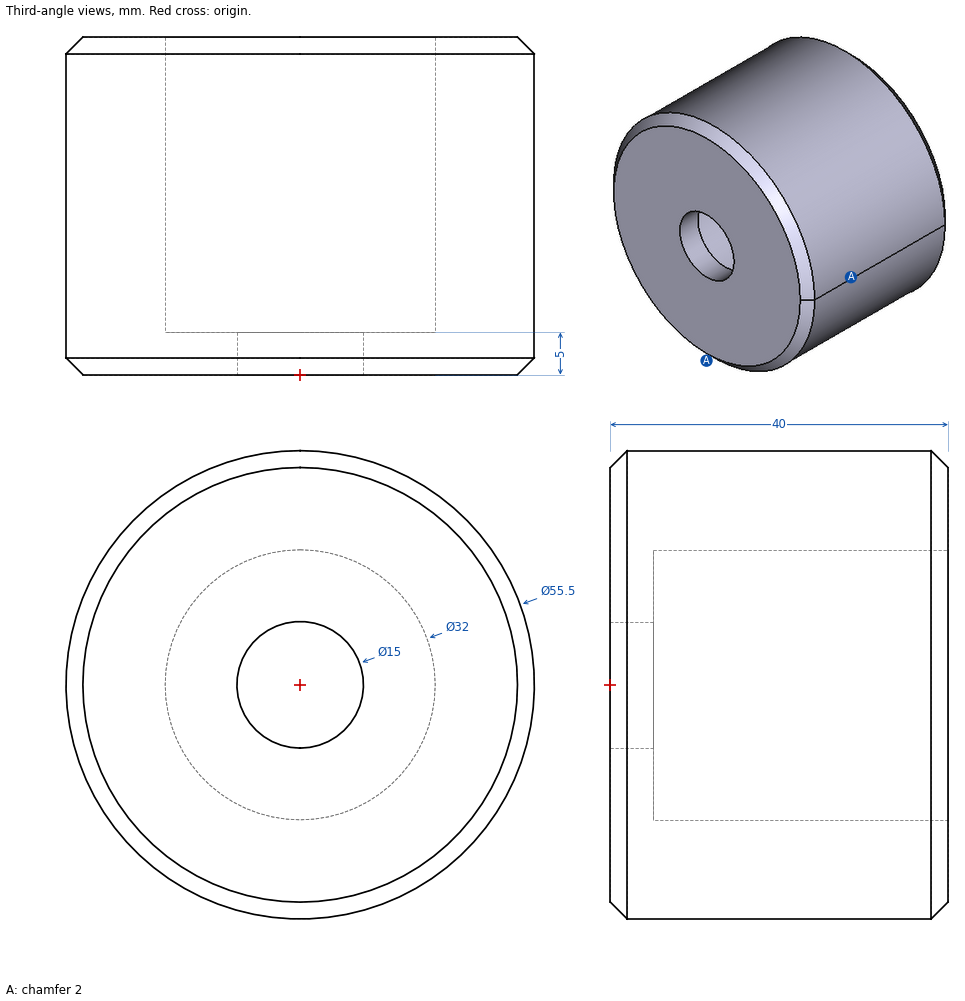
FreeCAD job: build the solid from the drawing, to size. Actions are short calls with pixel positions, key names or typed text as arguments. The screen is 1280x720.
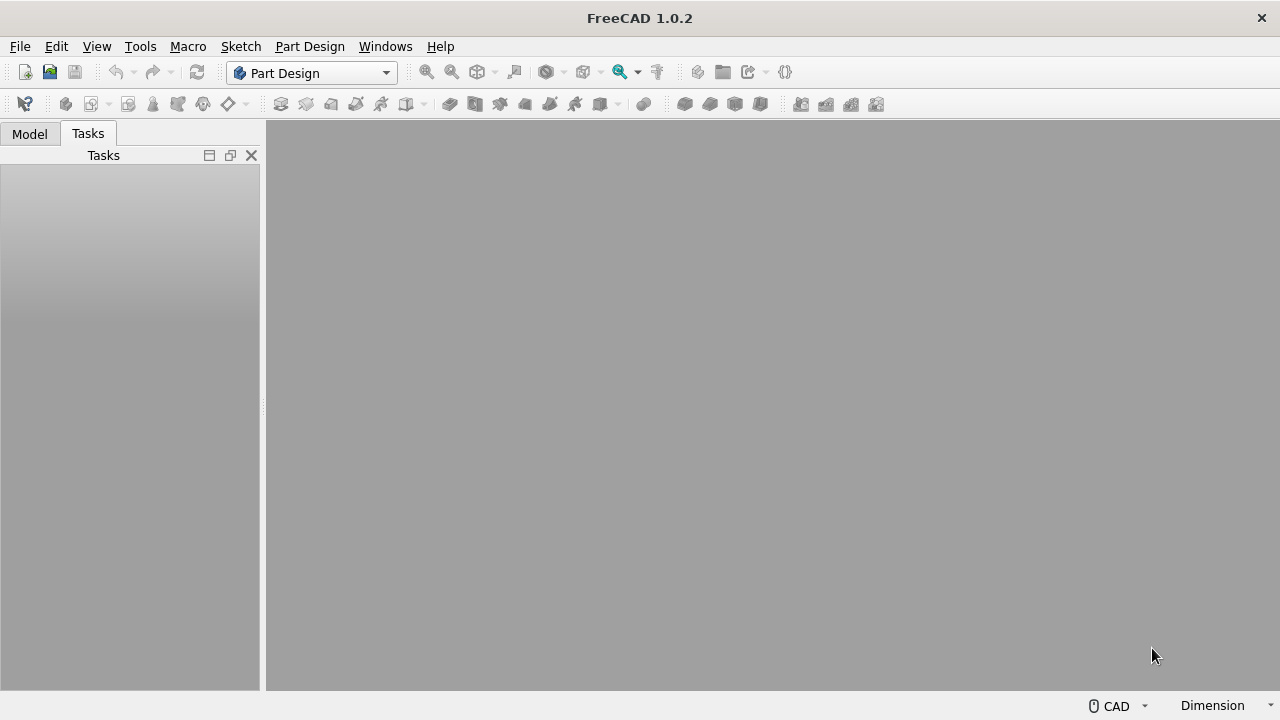
click(25, 72)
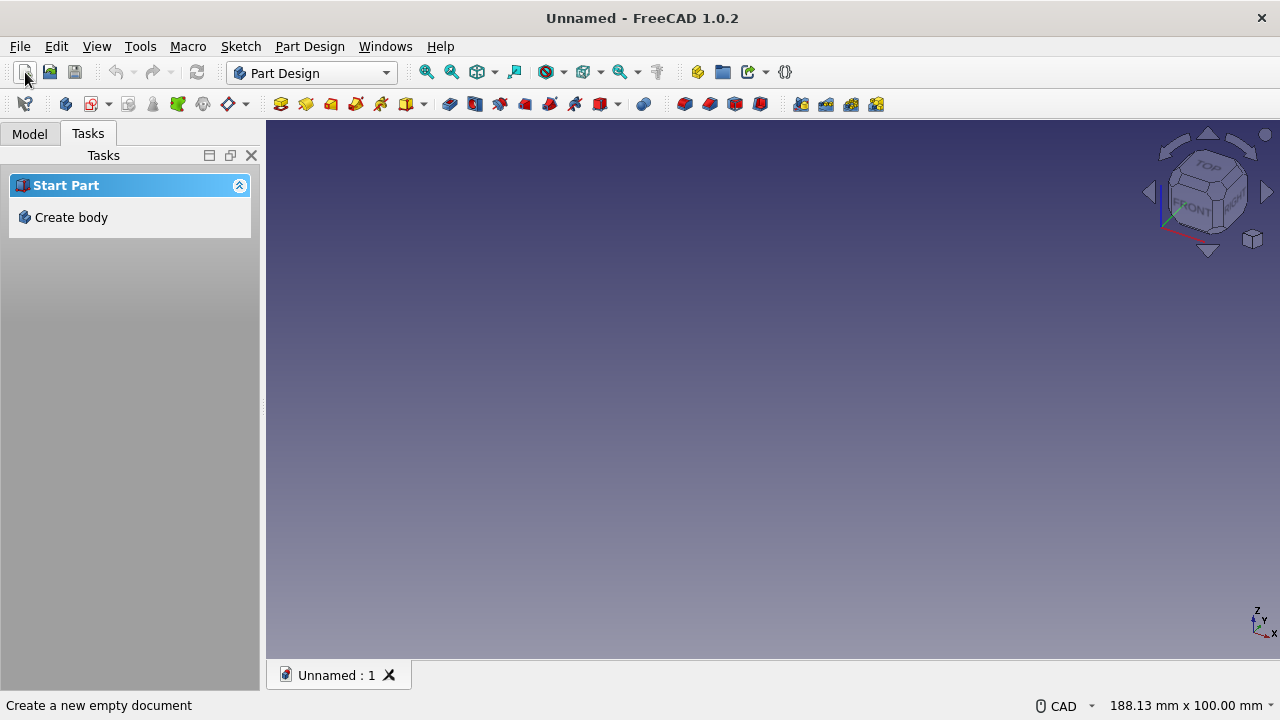
click(90, 104)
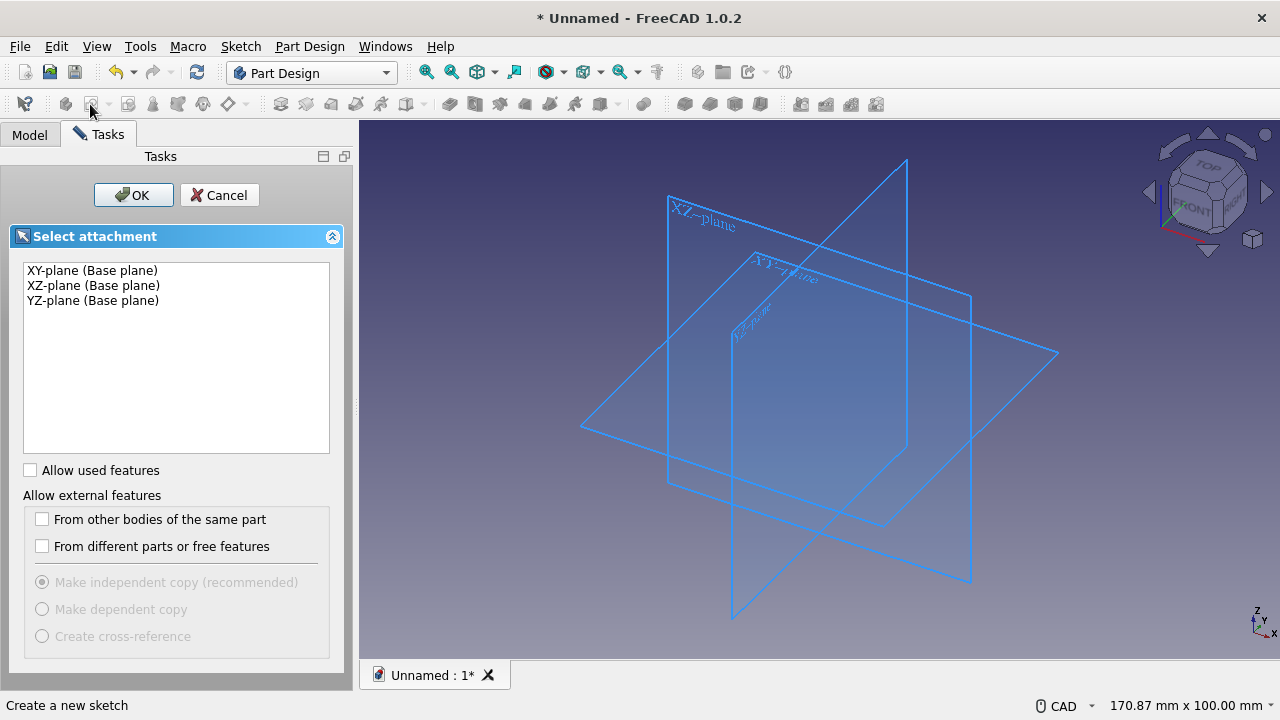
click(84, 286)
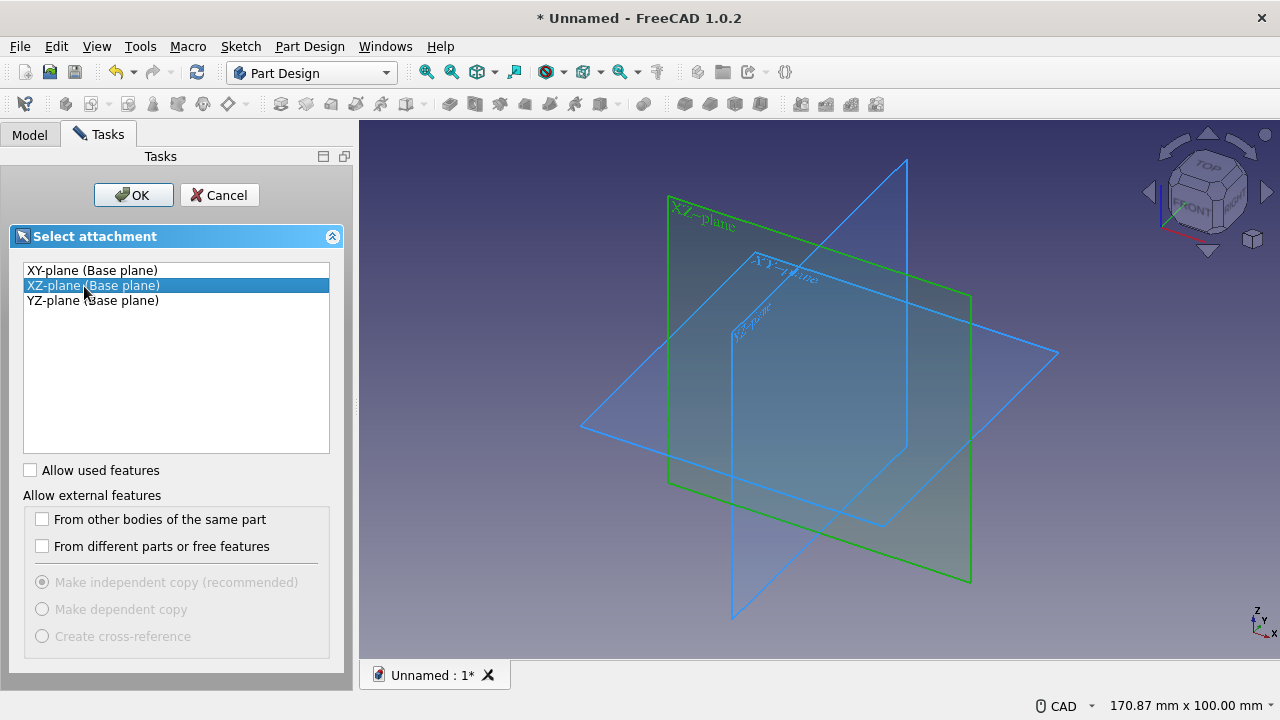
click(134, 195)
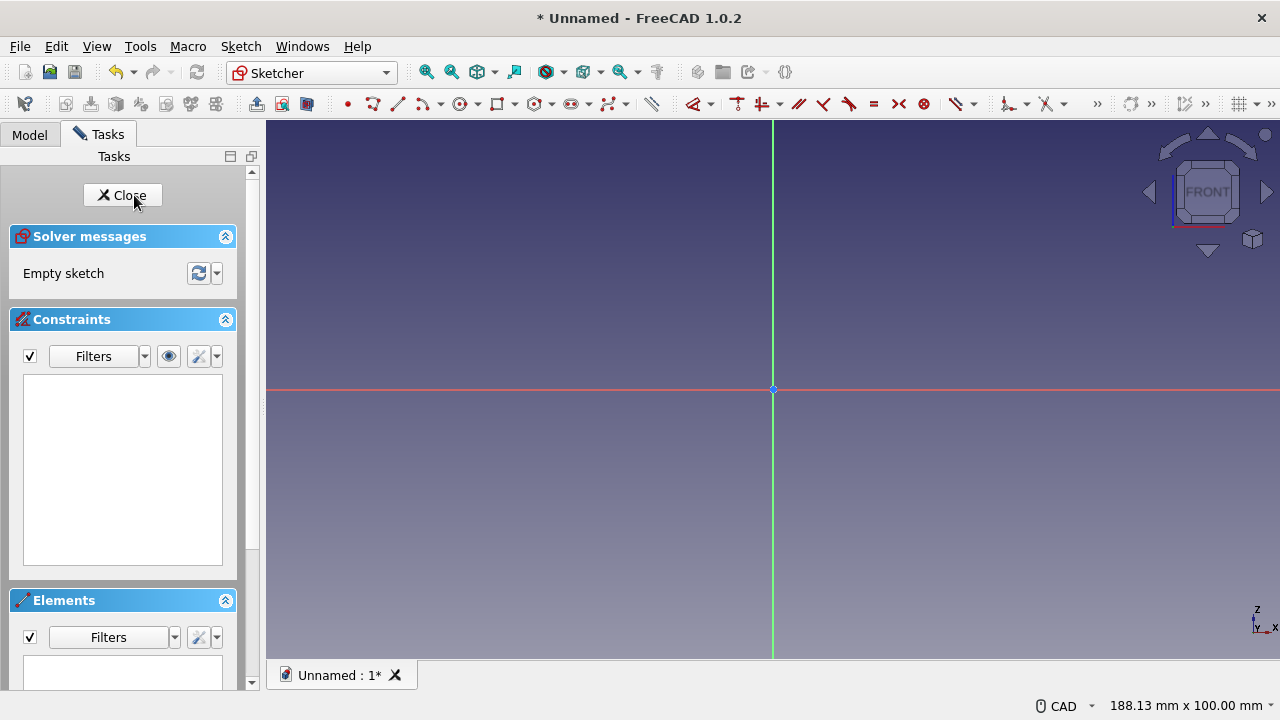
click(460, 104)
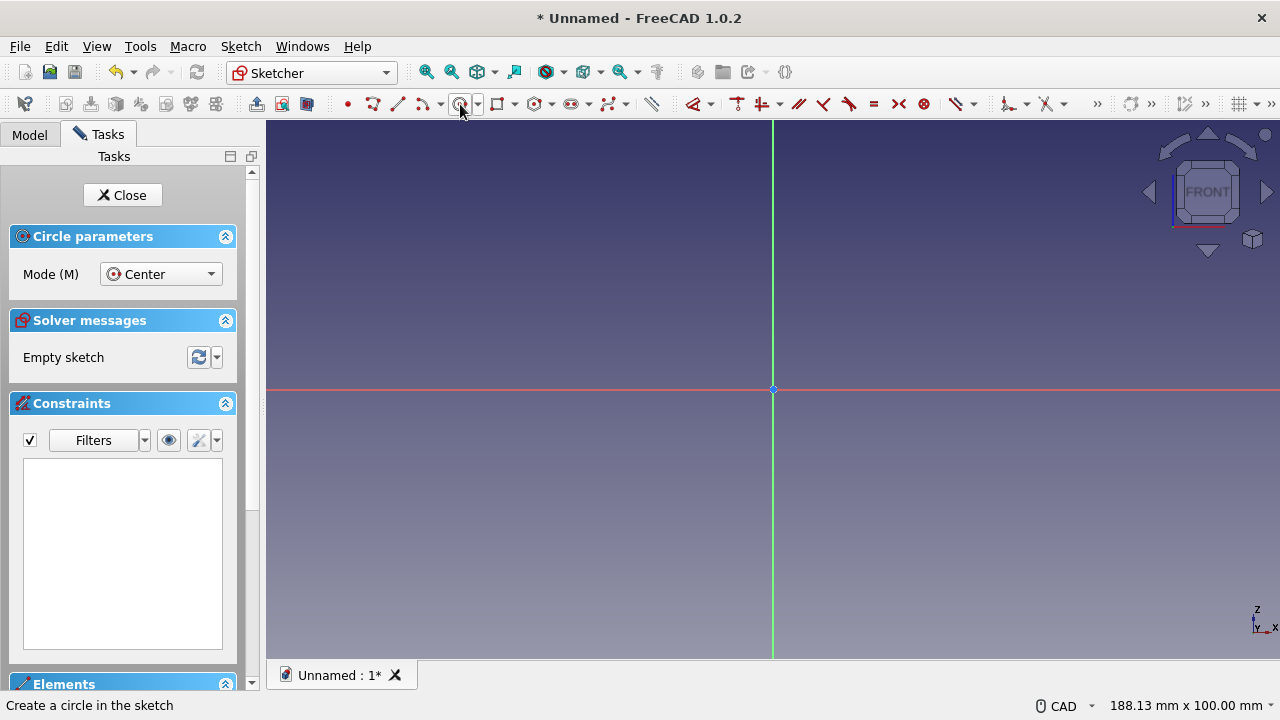
click(773, 390)
click(879, 284)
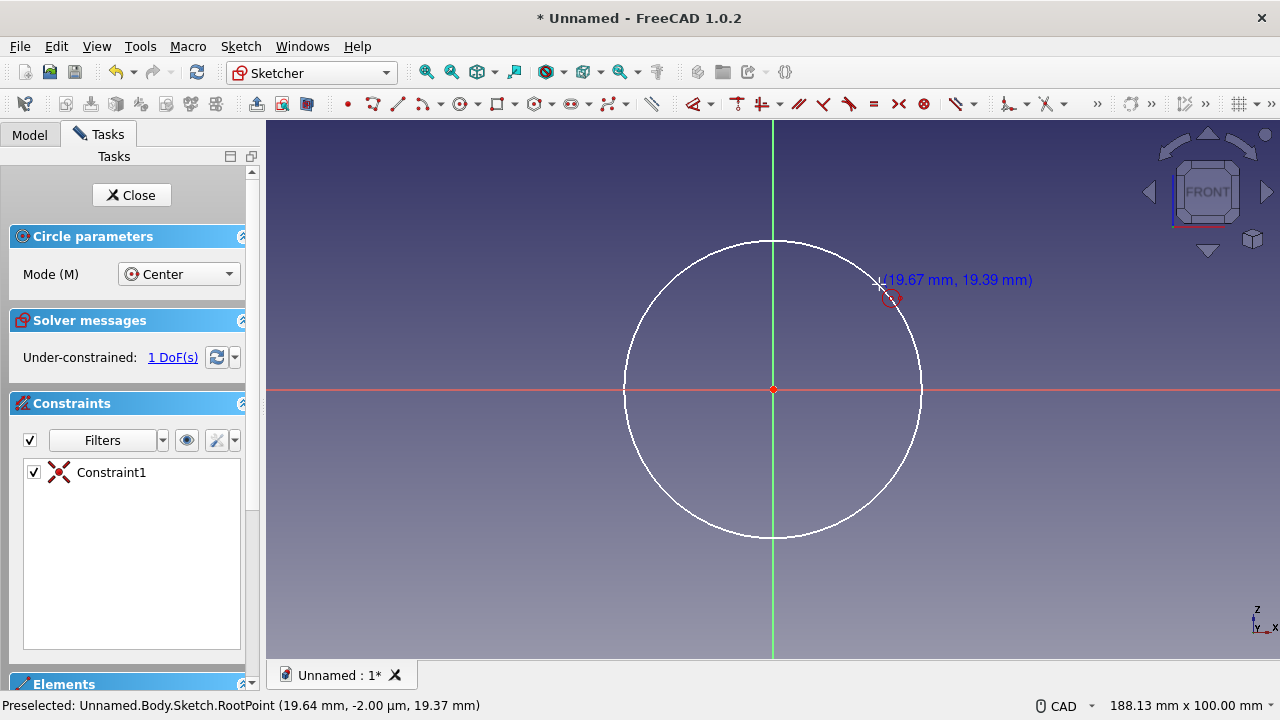
click(773, 390)
click(834, 329)
key(Escape)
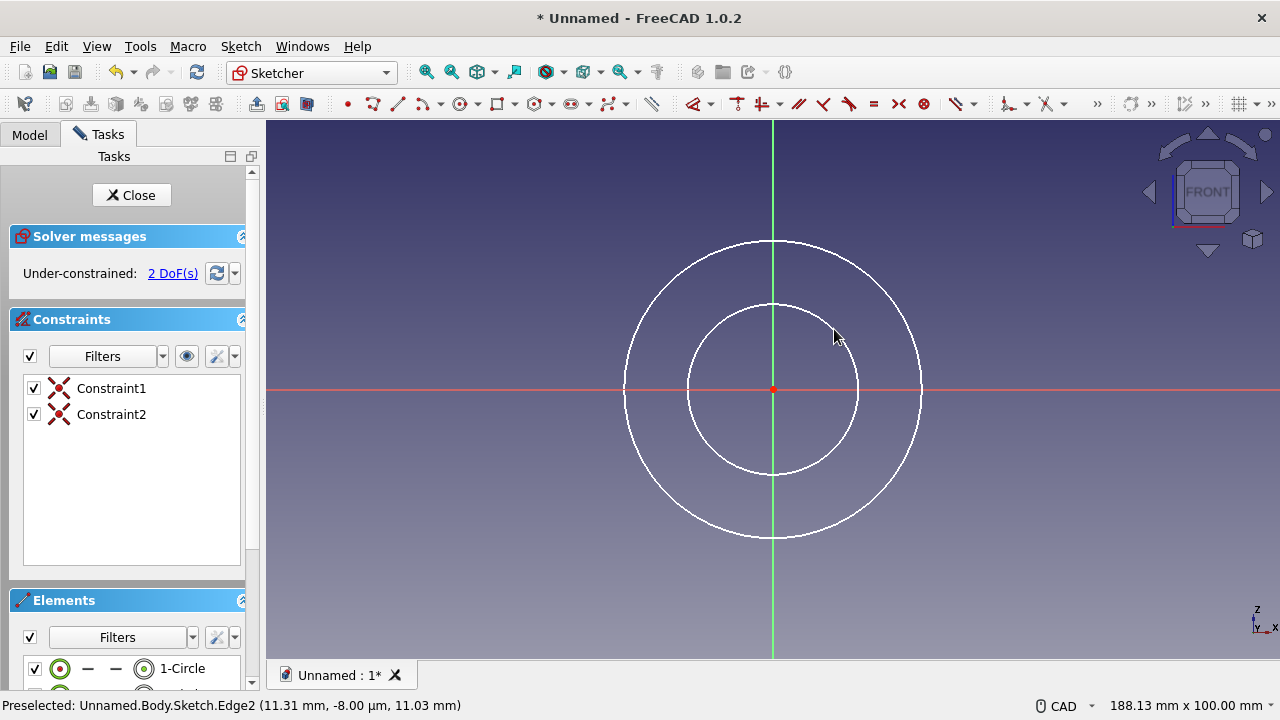
click(878, 284)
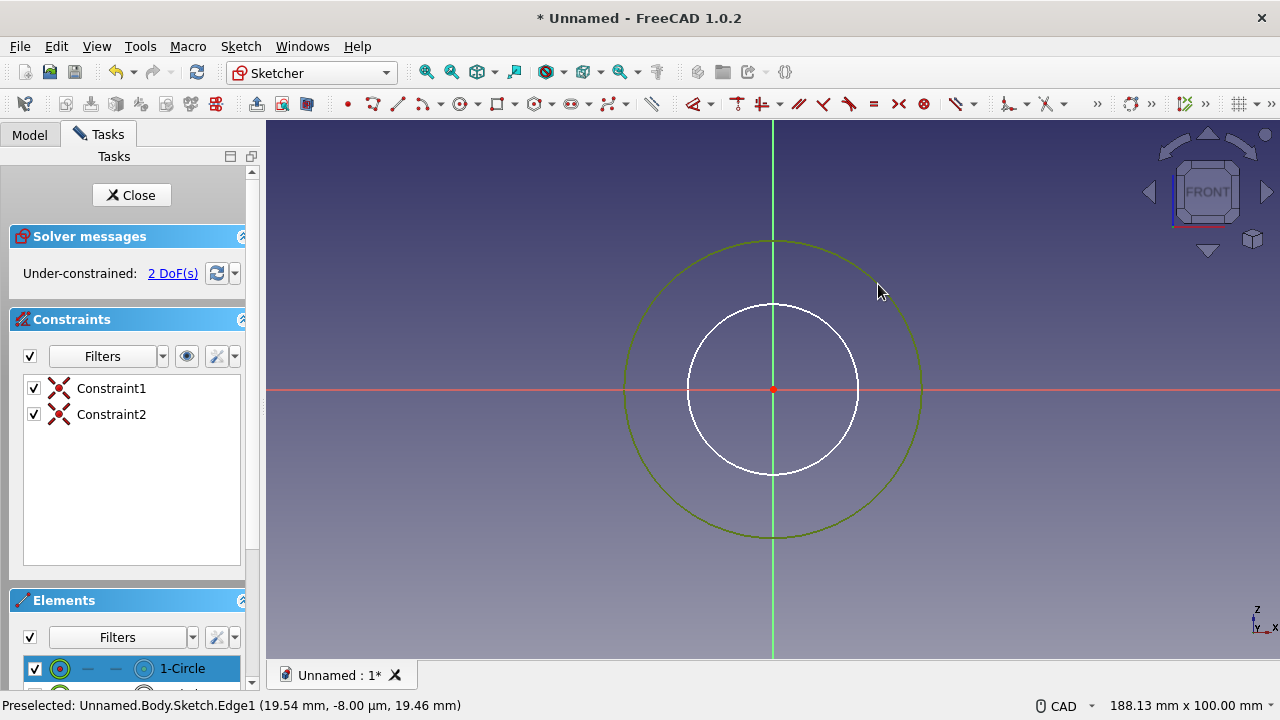
click(710, 104)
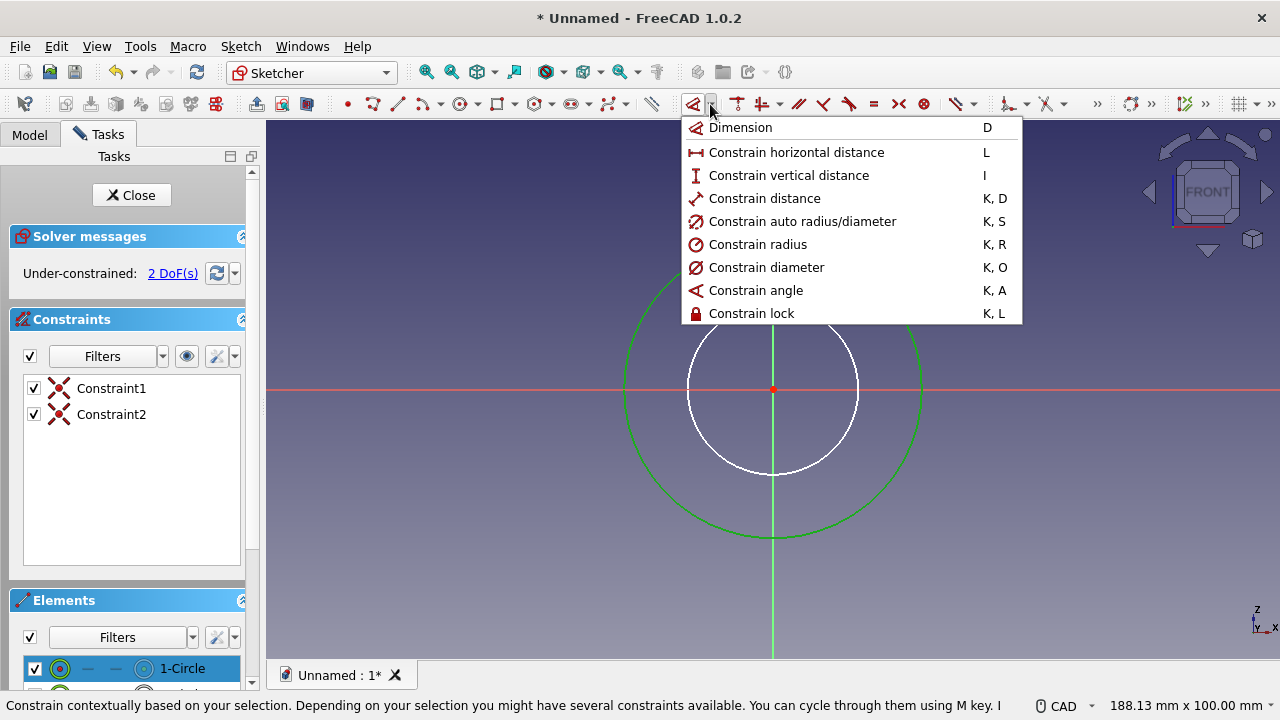
click(852, 268)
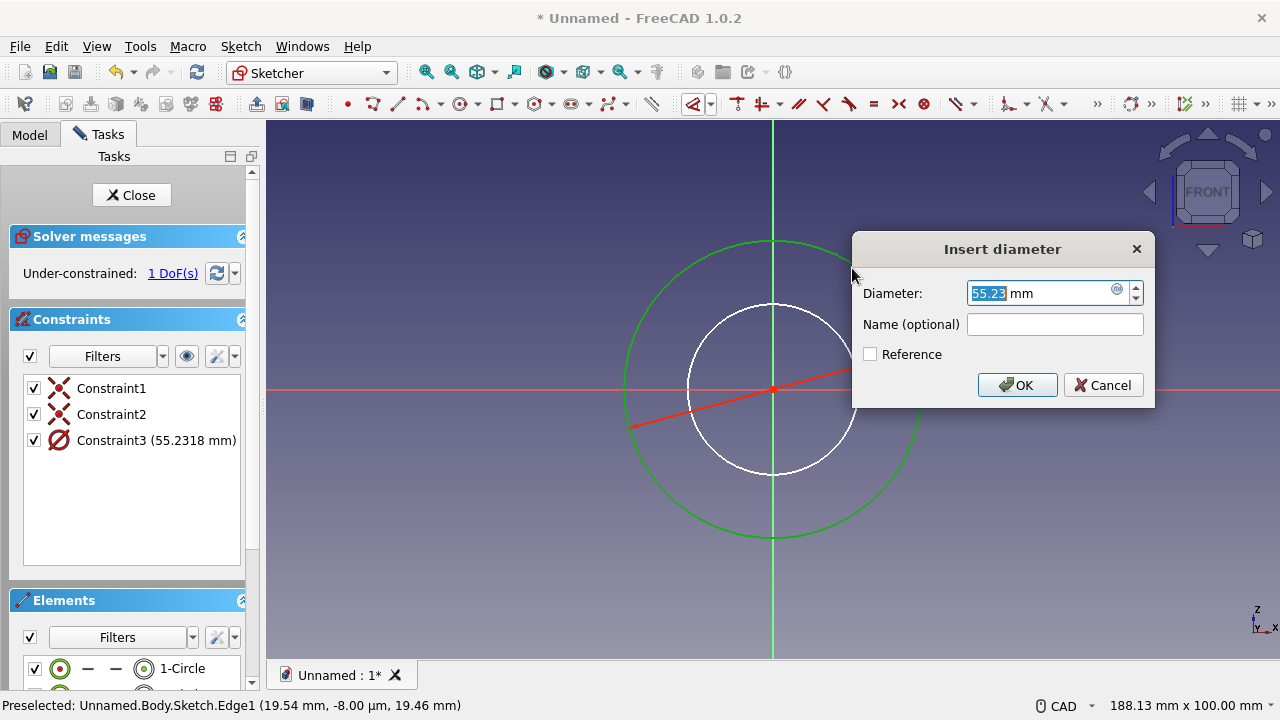
text(55.5)
key(Return)